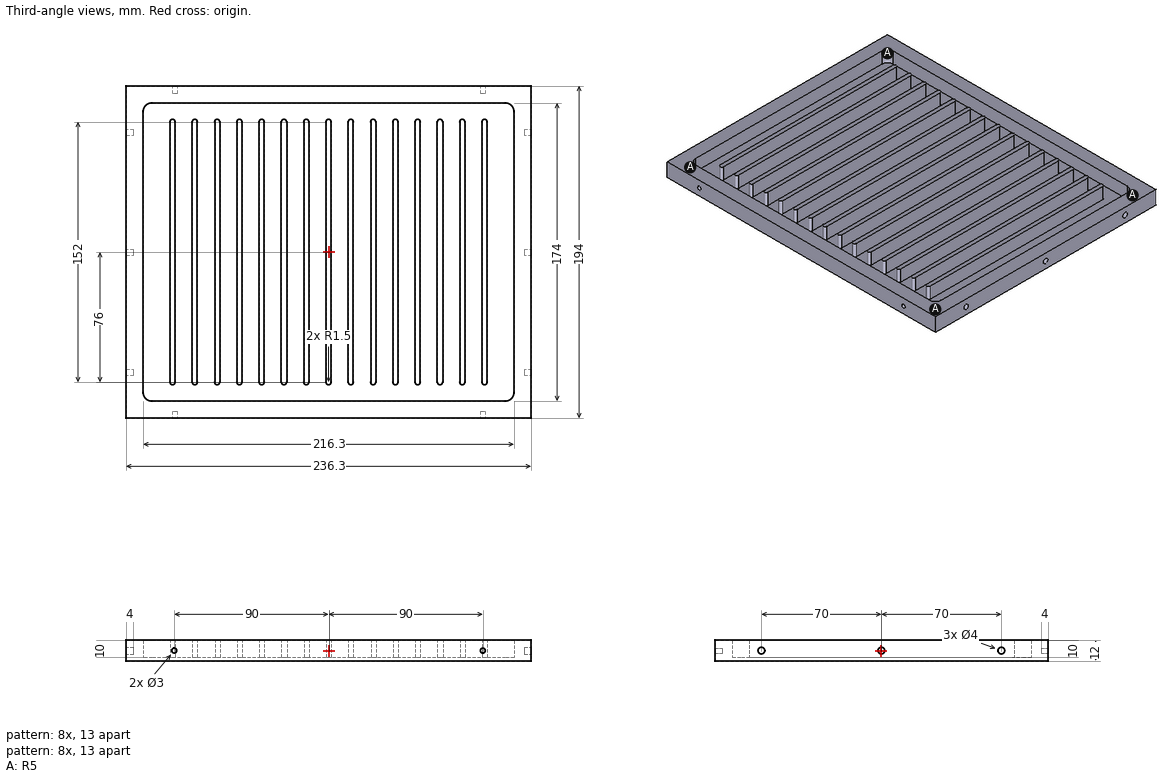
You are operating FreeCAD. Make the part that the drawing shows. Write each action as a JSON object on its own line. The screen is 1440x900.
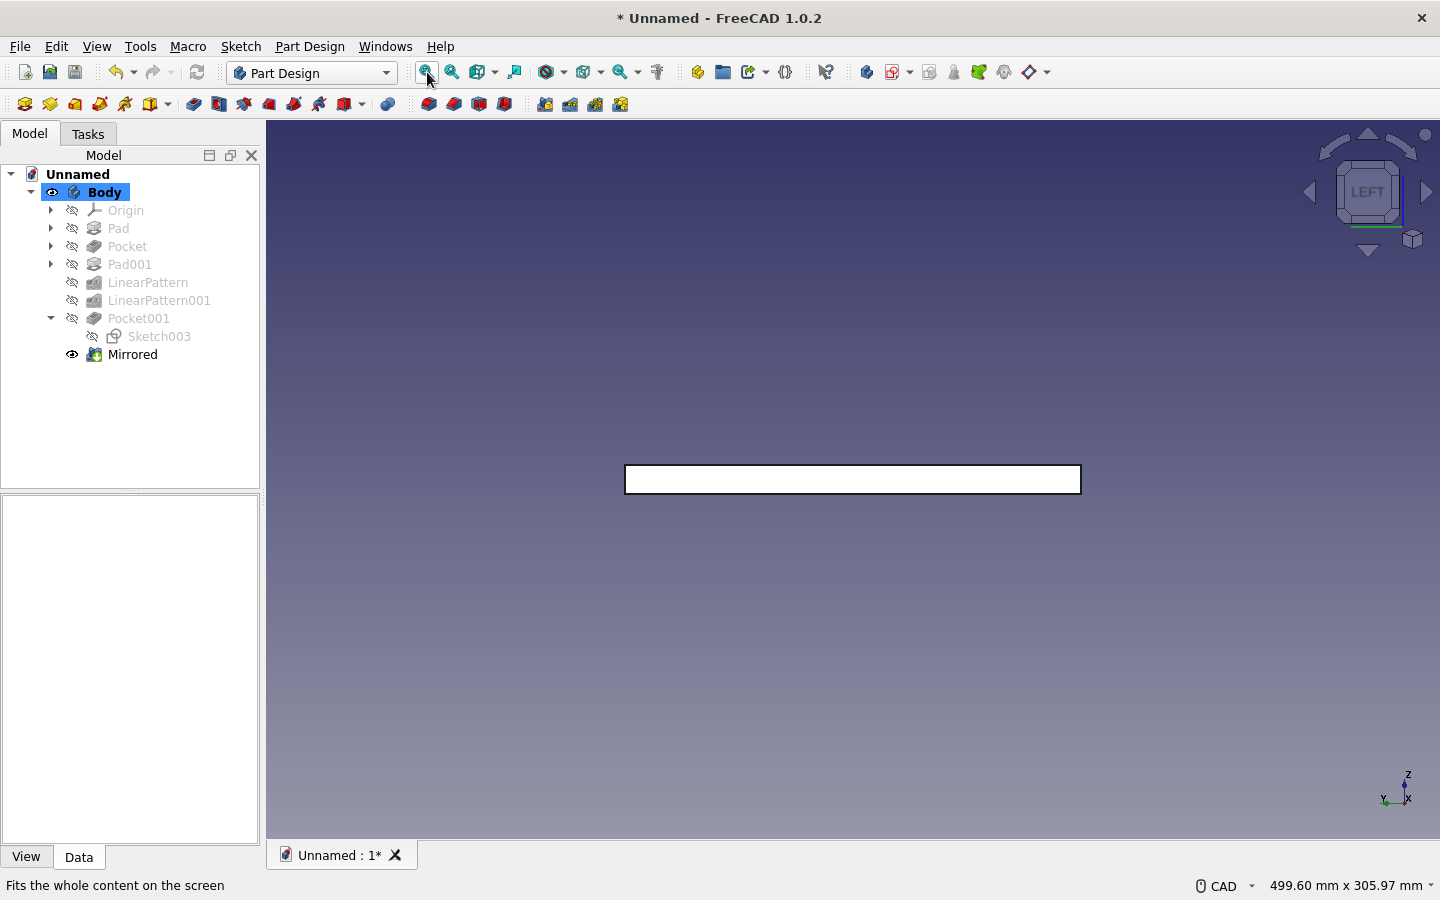
{"action": "left_click", "coordinate": [658, 478]}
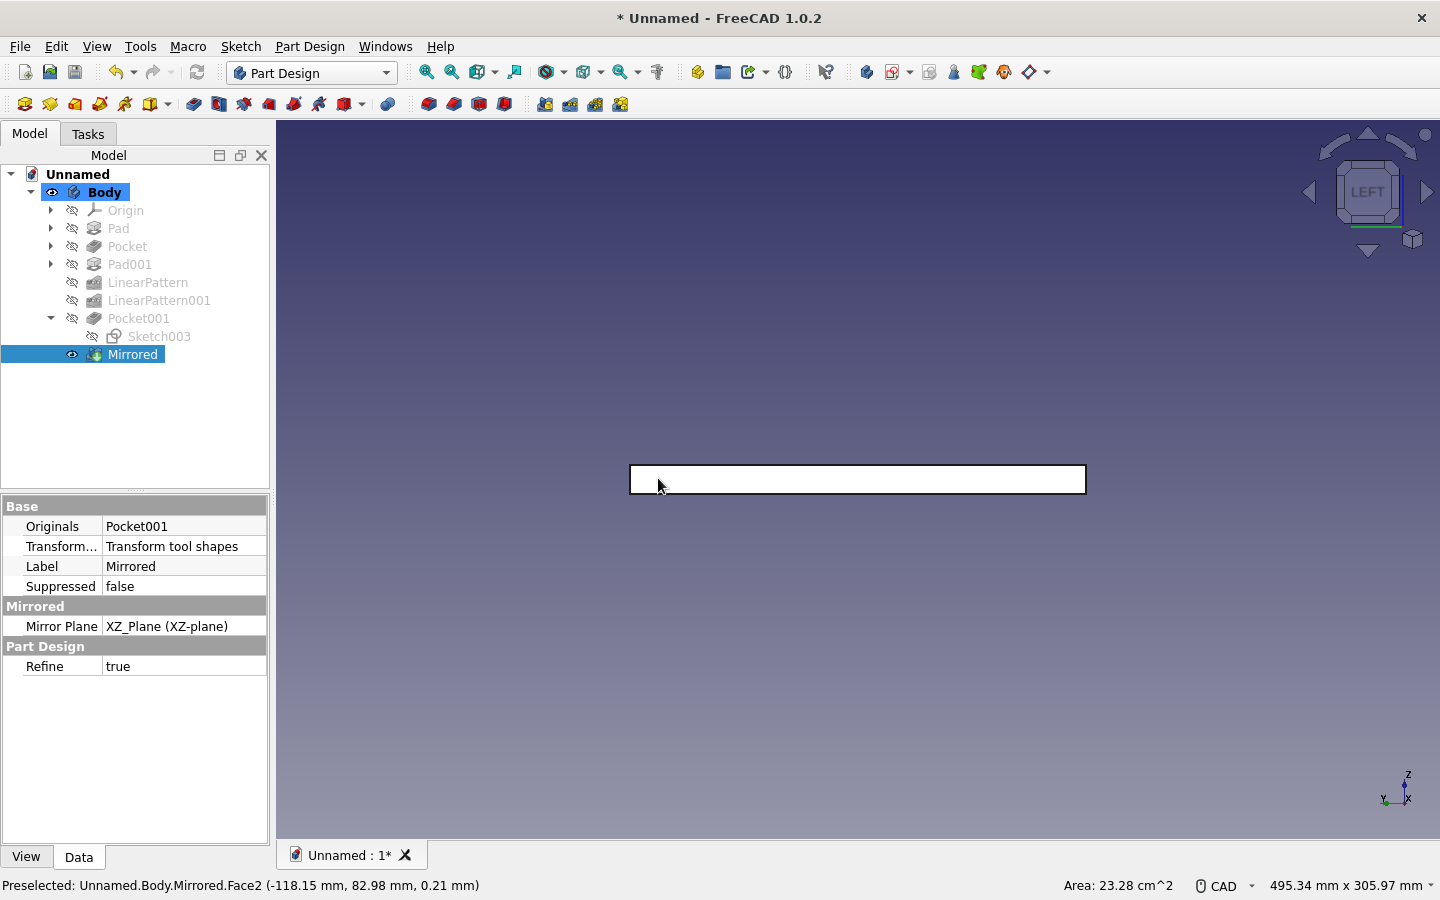
{"action": "left_click", "coordinate": [892, 72]}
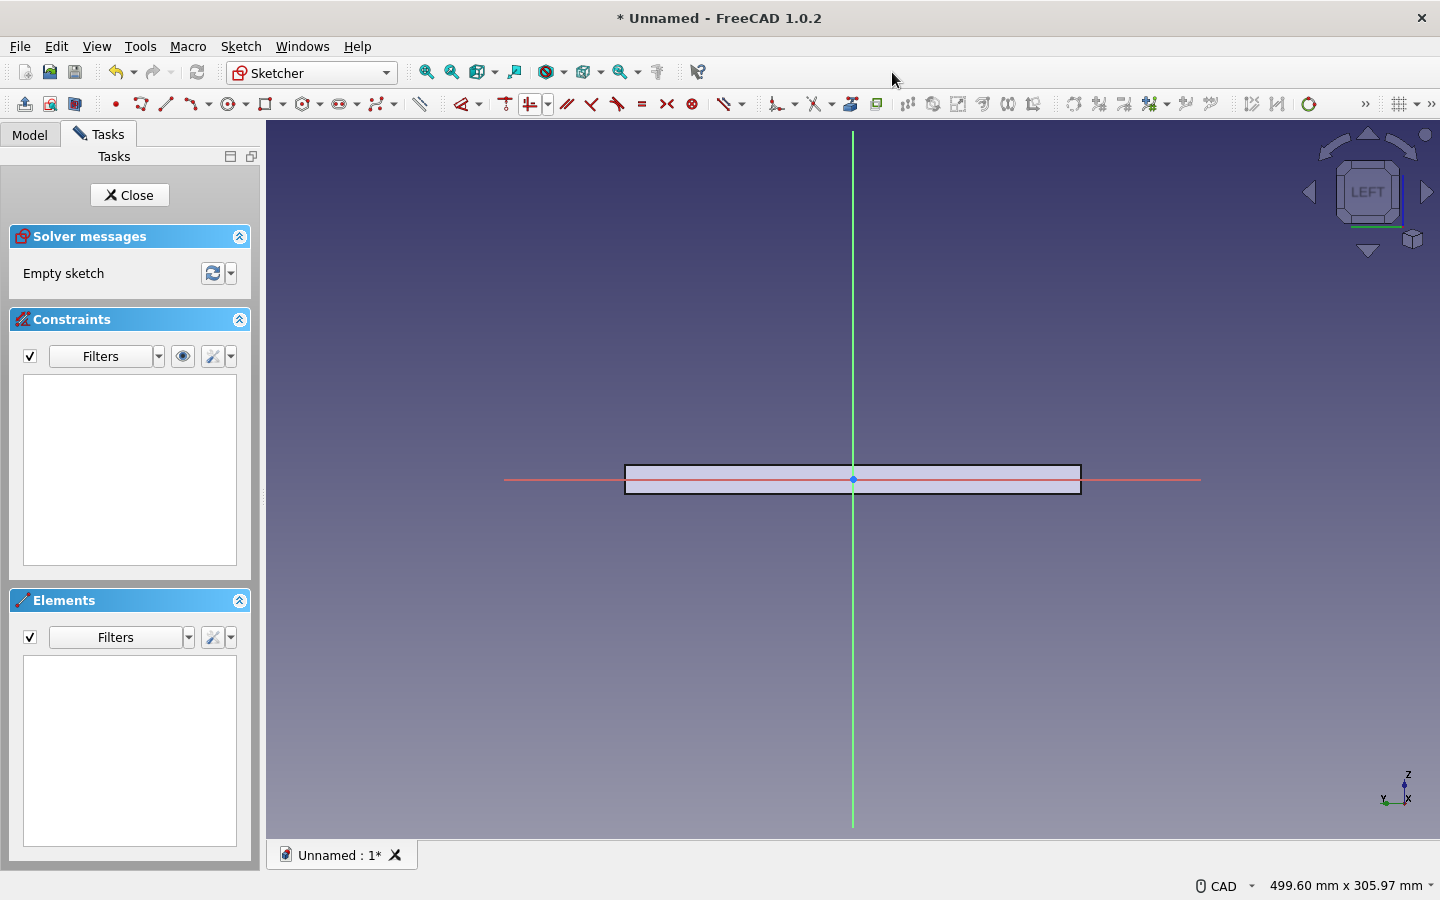
{"action": "scroll", "coordinate": [909, 480], "scroll_direction": "up", "scroll_amount": 4}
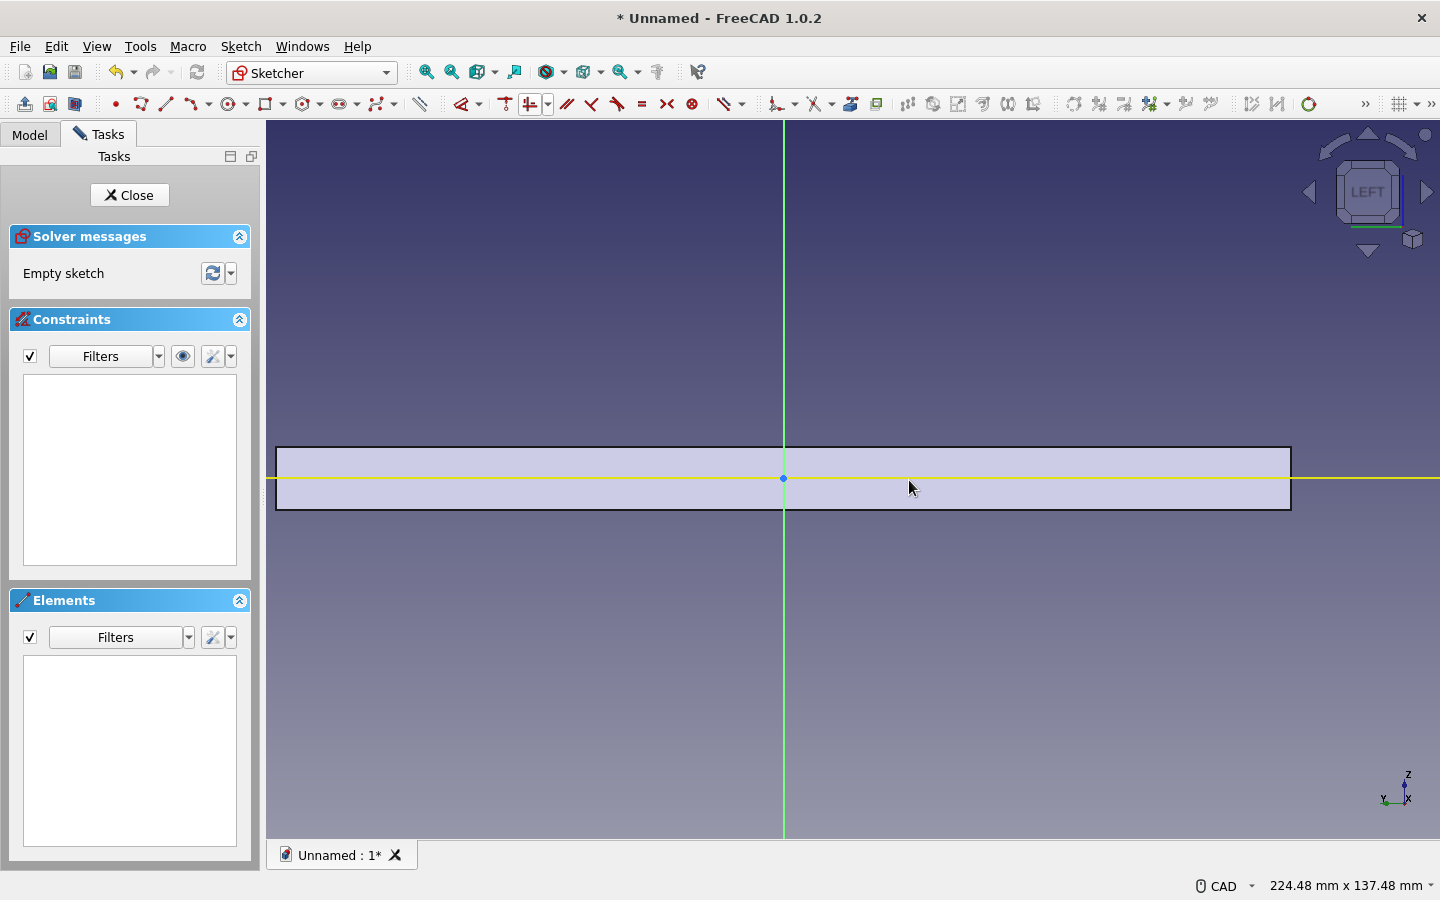
{"action": "left_click", "coordinate": [228, 104]}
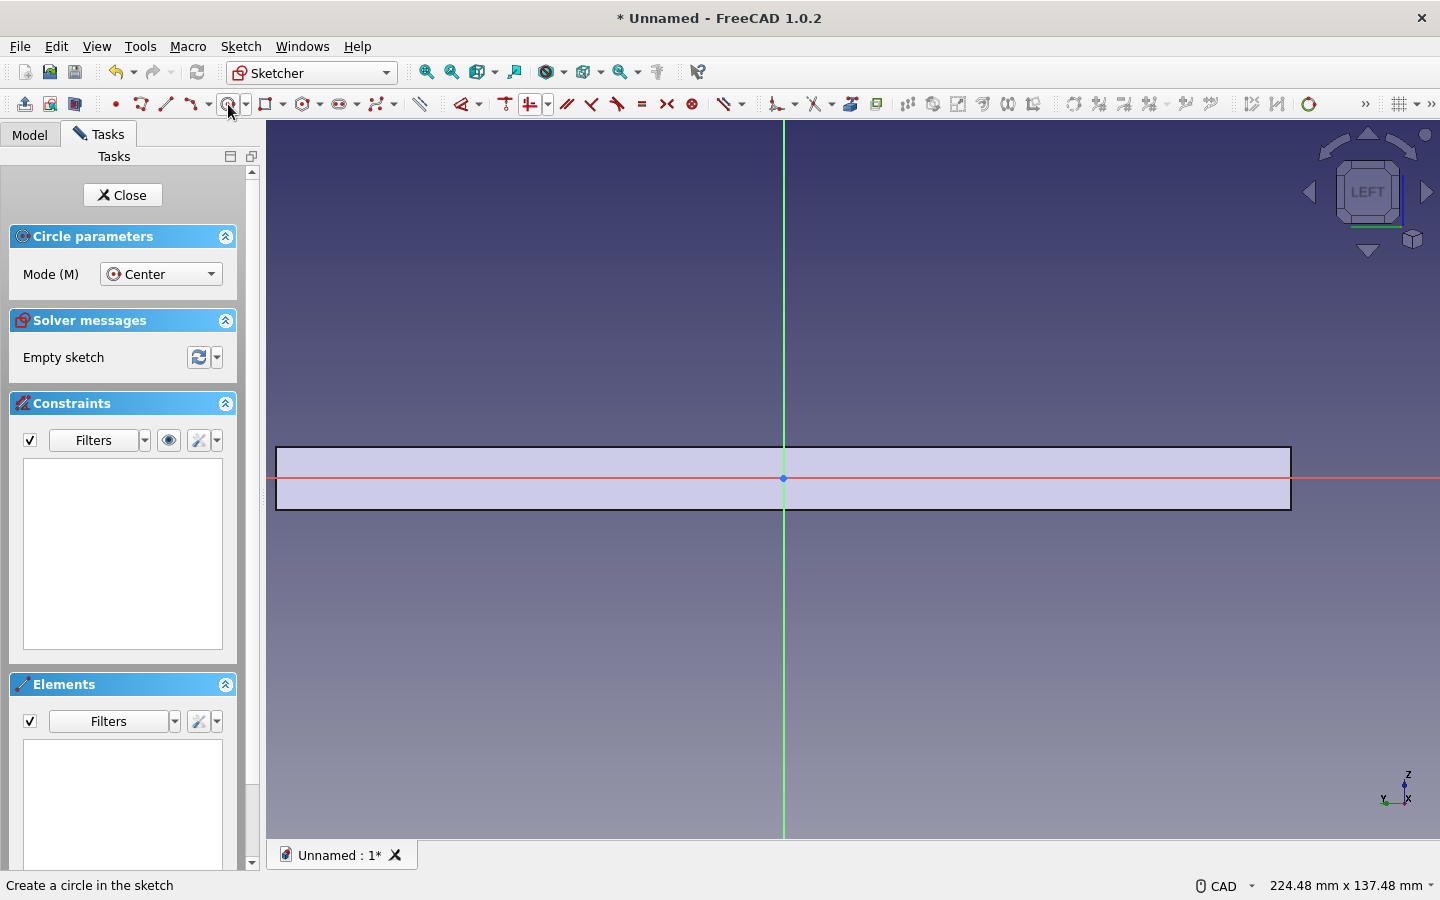
{"action": "scroll", "coordinate": [418, 478], "scroll_direction": "up", "scroll_amount": 4}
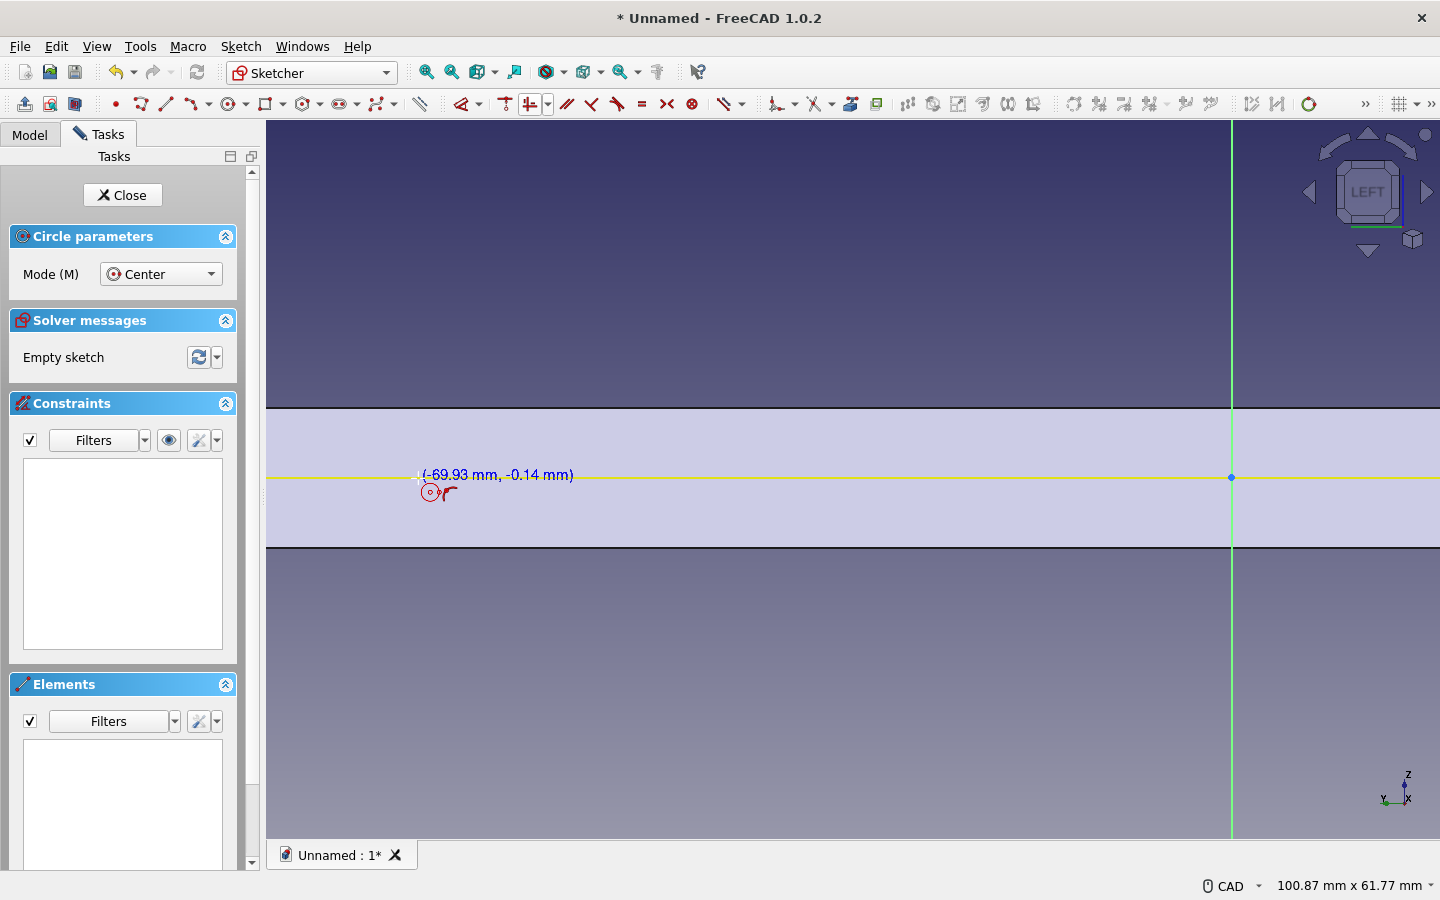
{"action": "left_click", "coordinate": [417, 478]}
{"action": "left_click", "coordinate": [433, 462]}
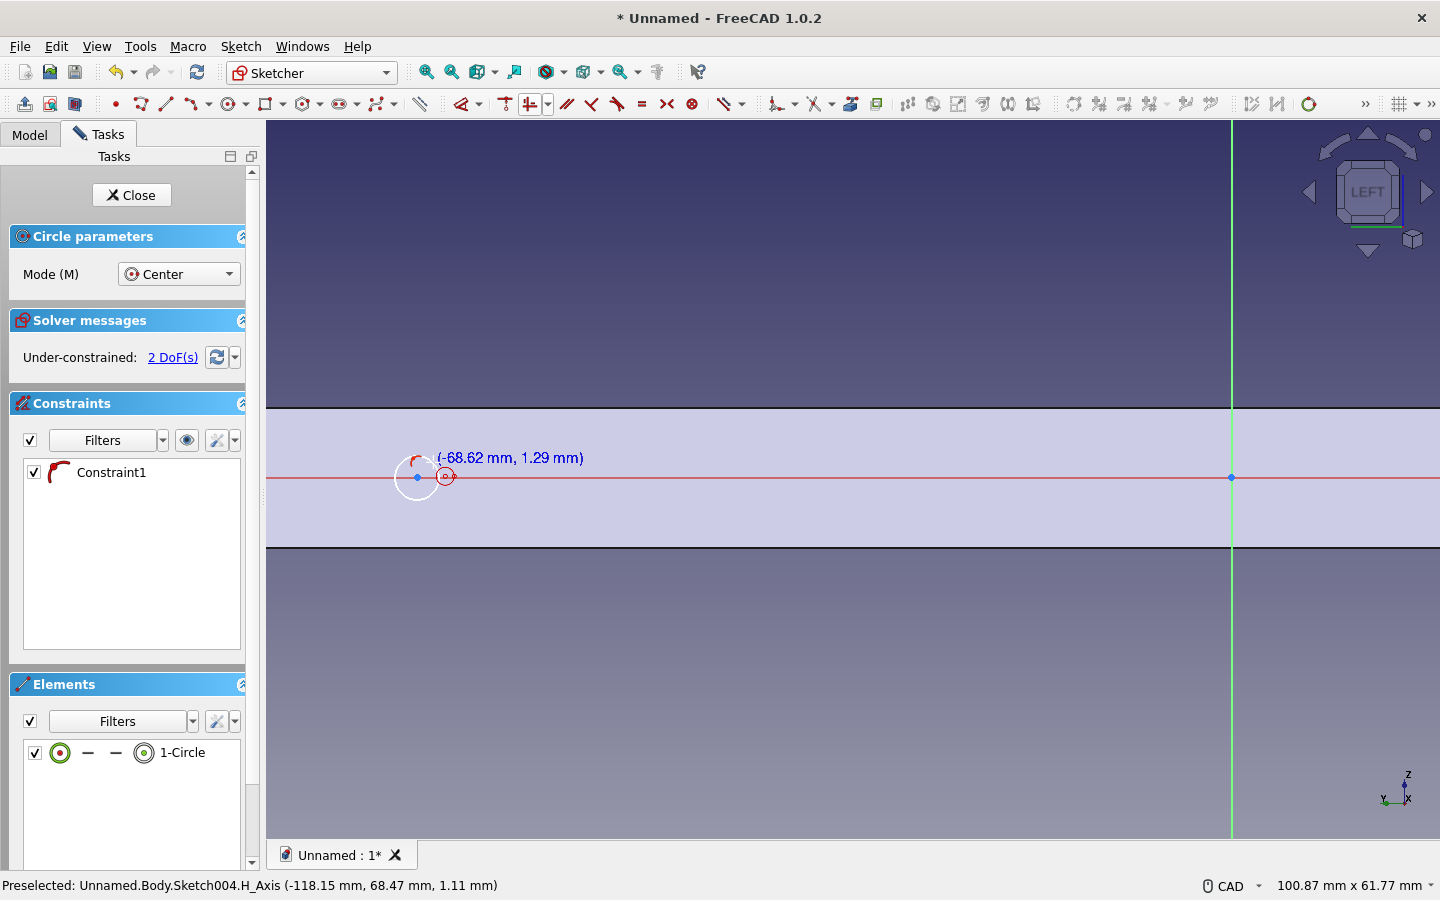
{"action": "left_click", "coordinate": [1232, 478]}
{"action": "left_click", "coordinate": [1248, 462]}